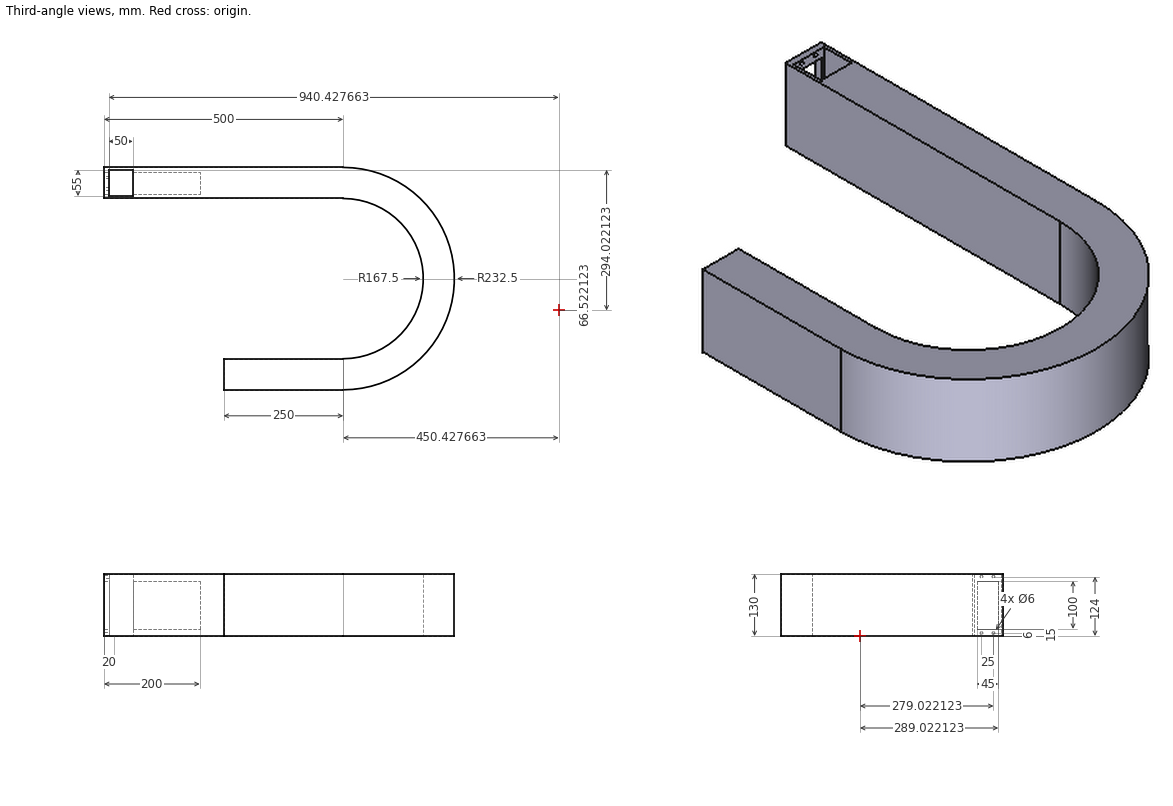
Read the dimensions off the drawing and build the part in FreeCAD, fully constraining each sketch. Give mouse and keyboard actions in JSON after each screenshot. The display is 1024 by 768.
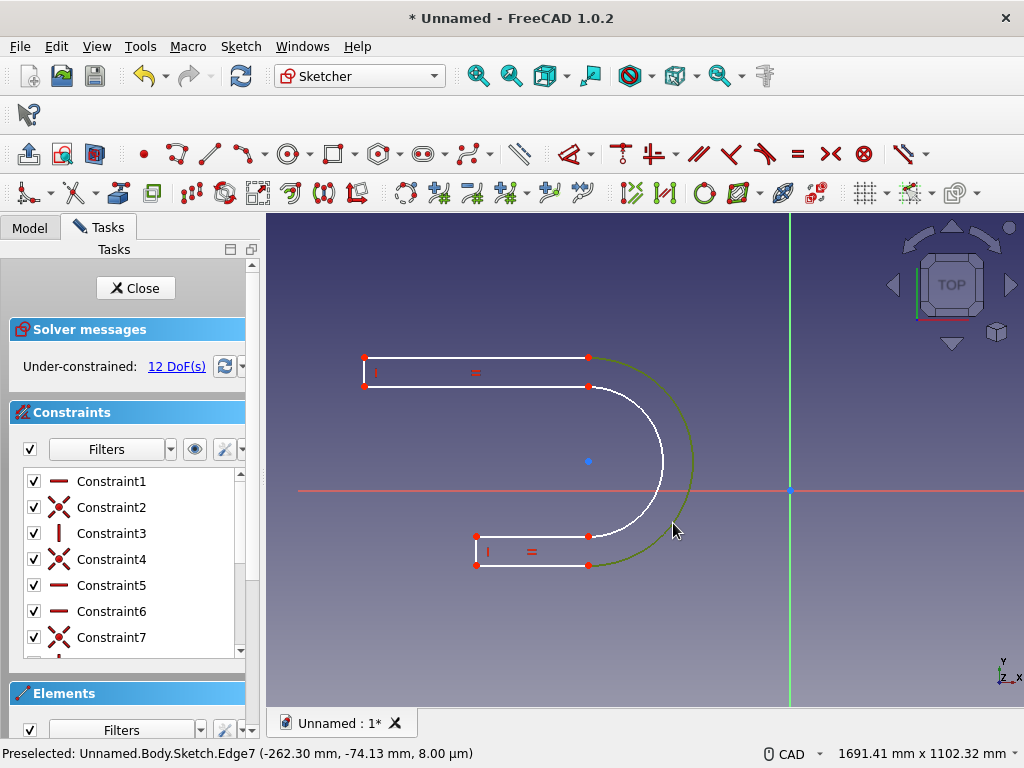
{"action": "left_click", "coordinate": [649, 506]}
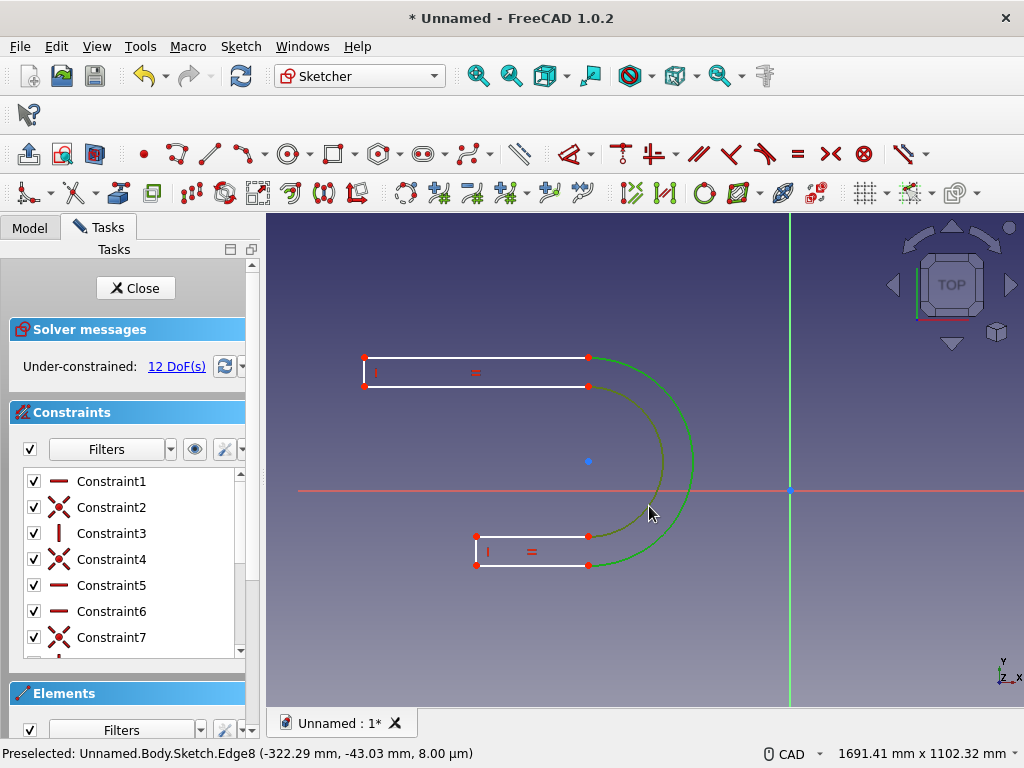
{"action": "left_click", "coordinate": [621, 154]}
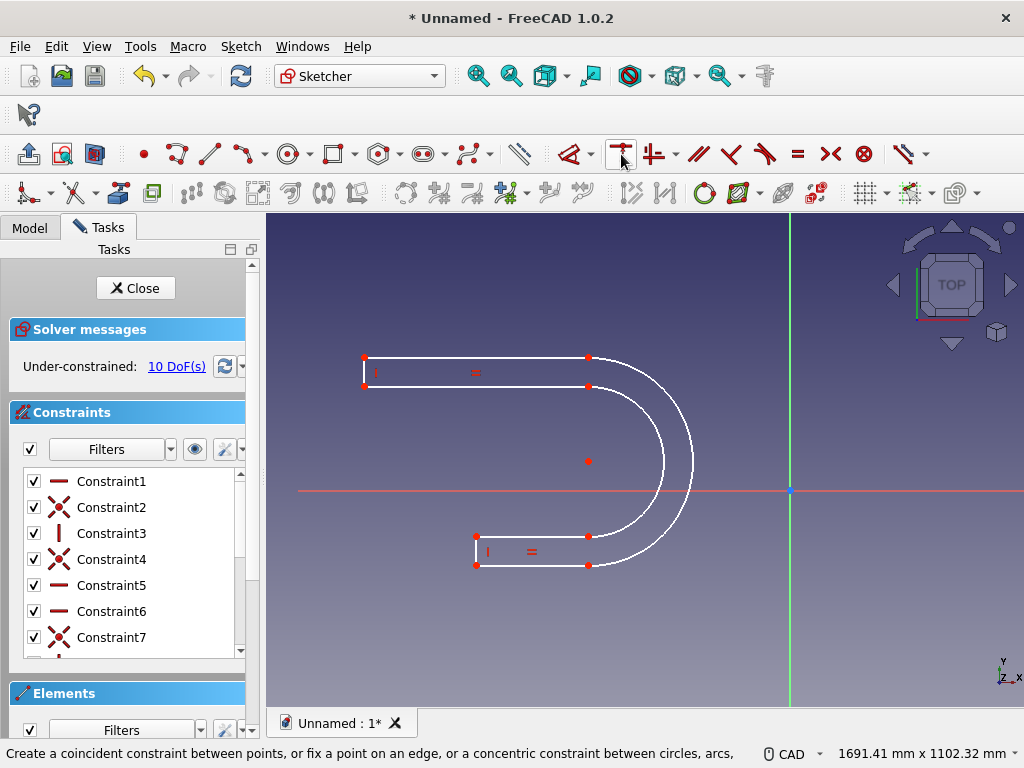
{"action": "left_click", "coordinate": [568, 154]}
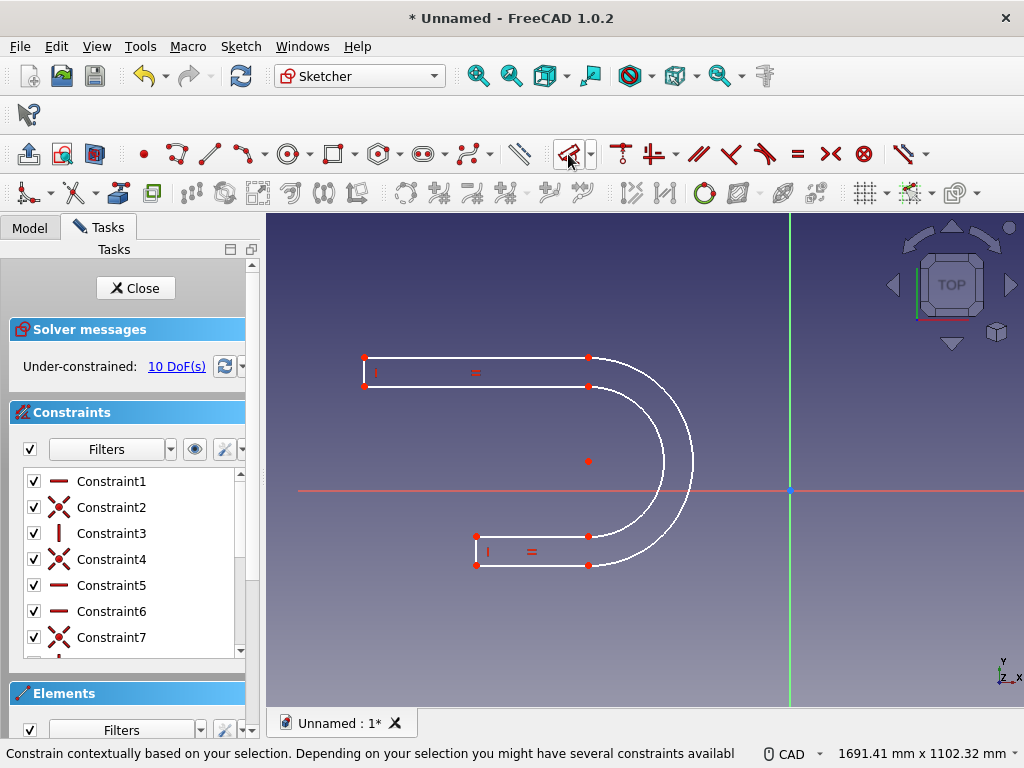
{"action": "left_click", "coordinate": [673, 523]}
{"action": "left_click", "coordinate": [699, 542]}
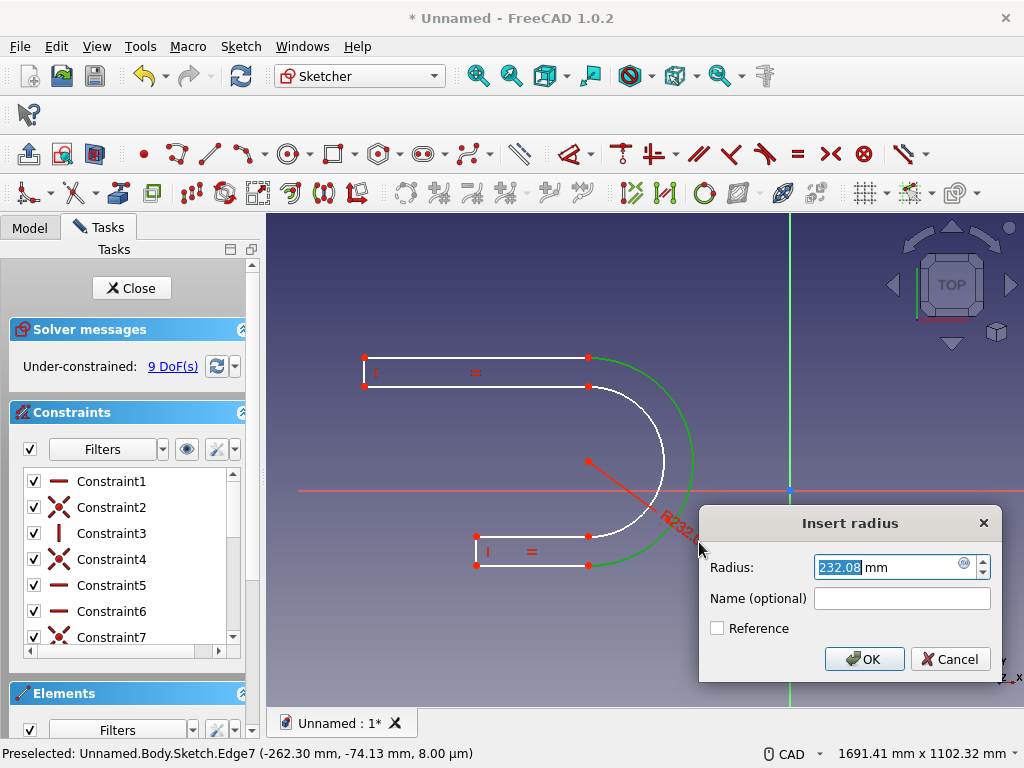
{"action": "type", "text": "232.5"}
{"action": "key", "text": "Return"}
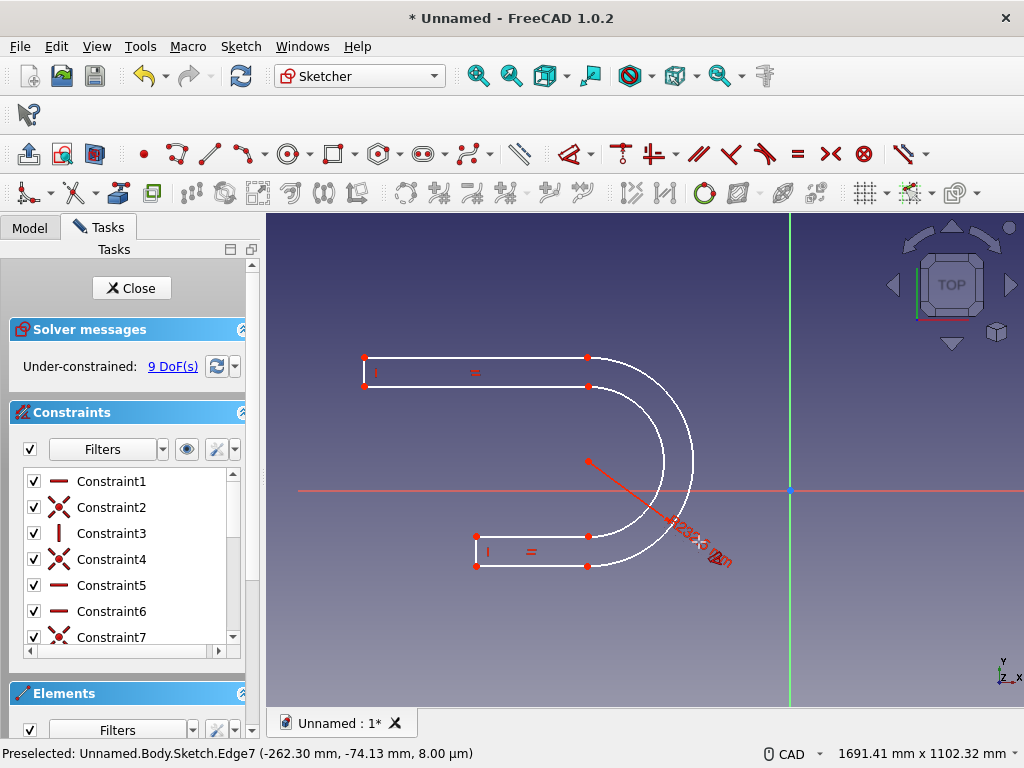
{"action": "left_click", "coordinate": [649, 506]}
{"action": "left_click", "coordinate": [644, 579]}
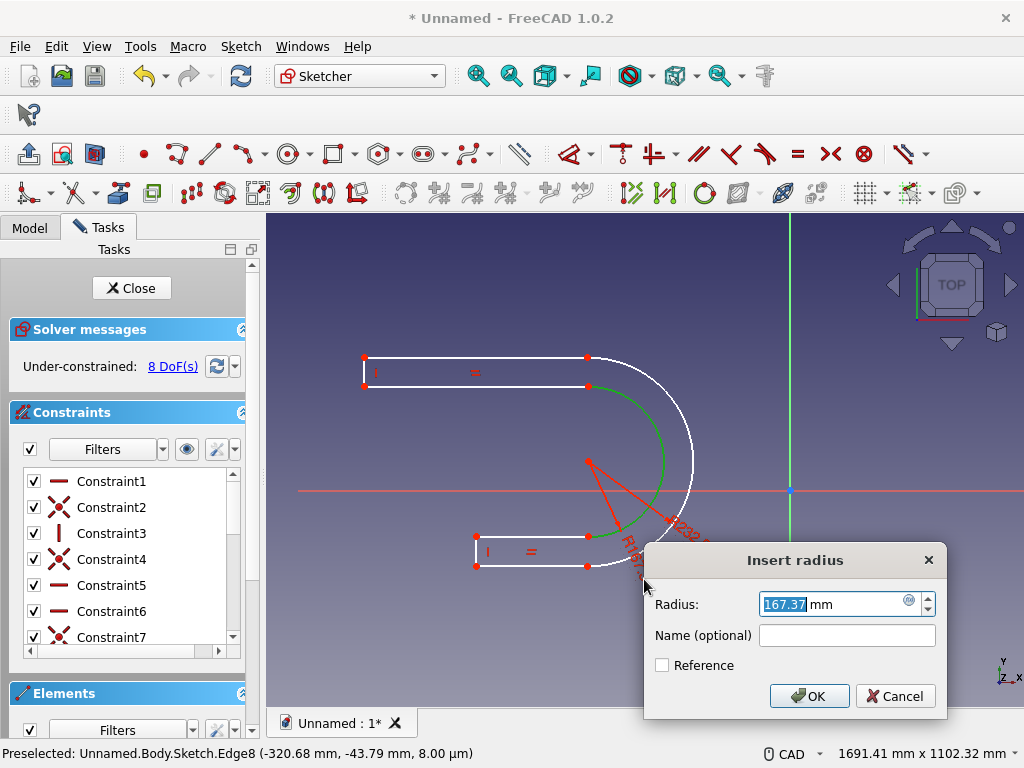
{"action": "type", "text": "167.5"}
{"action": "key", "text": "Return"}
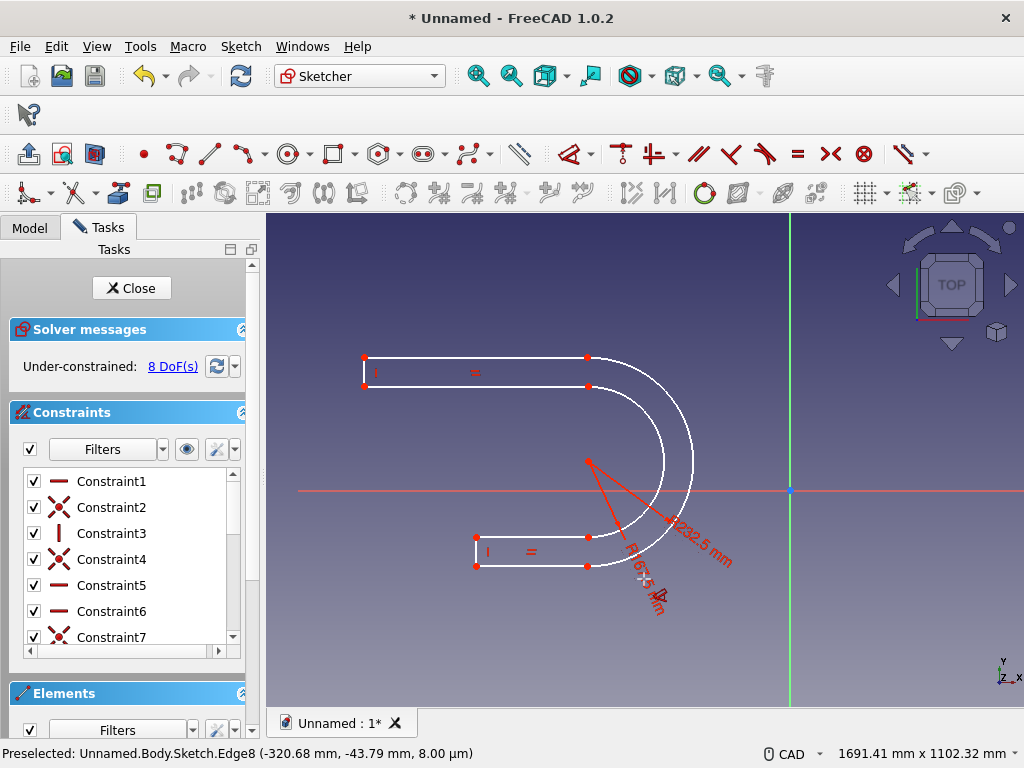
{"action": "left_click", "coordinate": [554, 537]}
{"action": "left_click", "coordinate": [532, 595]}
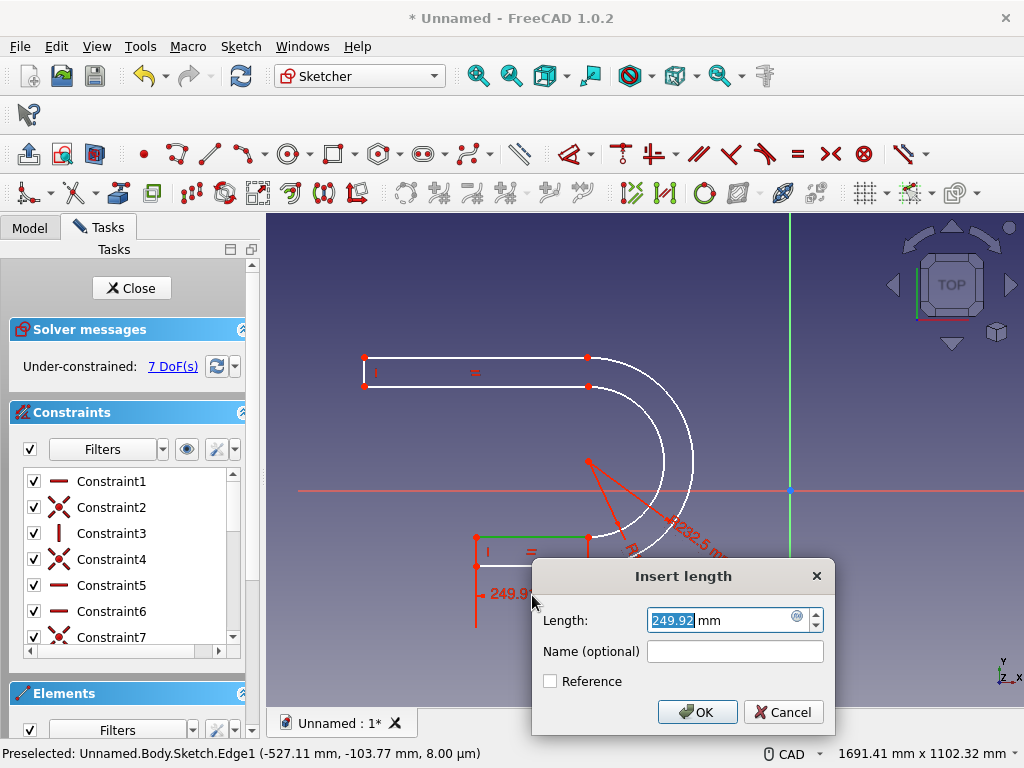
{"action": "type", "text": "250"}
{"action": "key", "text": "Return"}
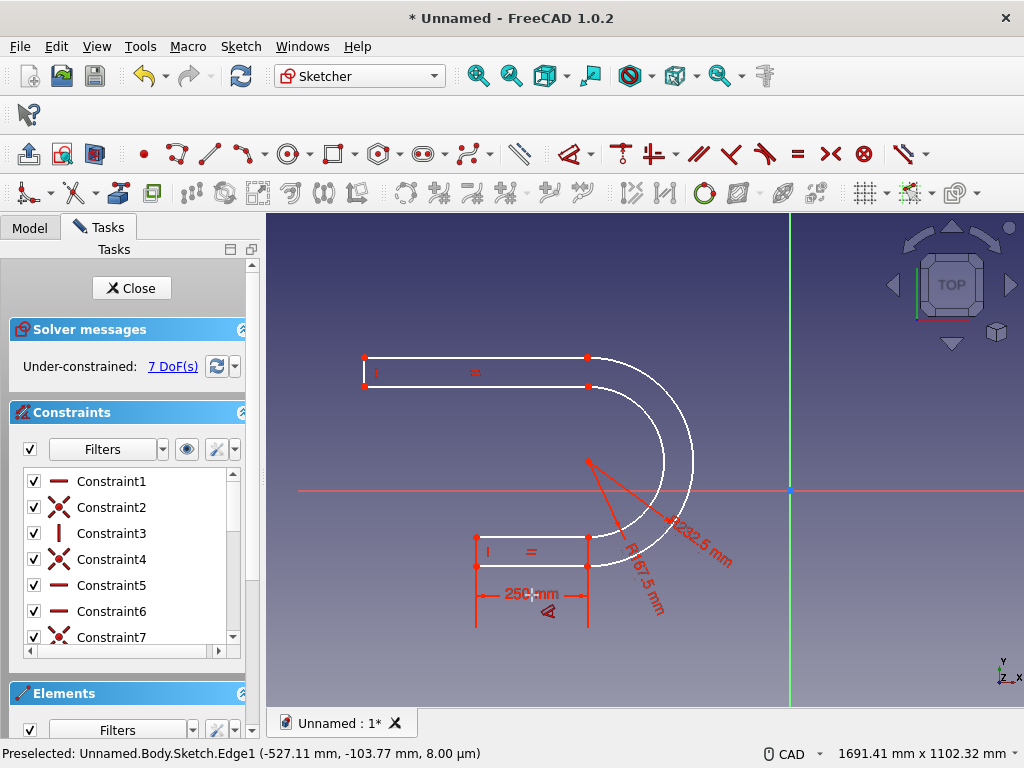
{"action": "left_click", "coordinate": [510, 566]}
{"action": "left_click", "coordinate": [532, 624]}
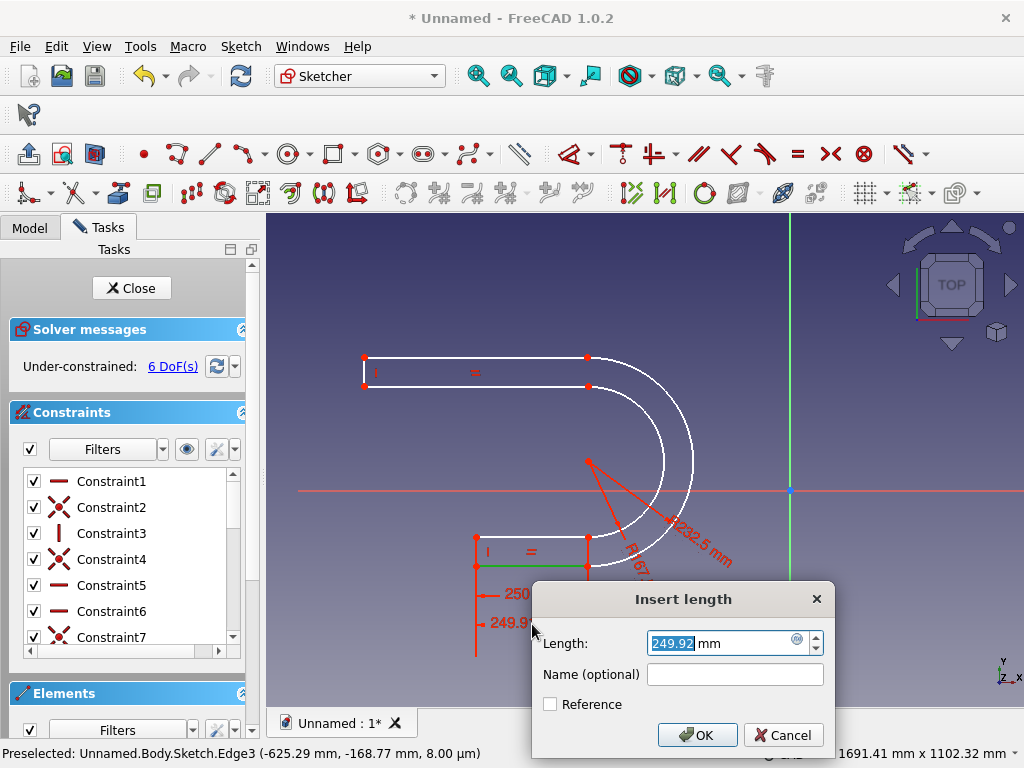
{"action": "type", "text": "250"}
{"action": "key", "text": "Return"}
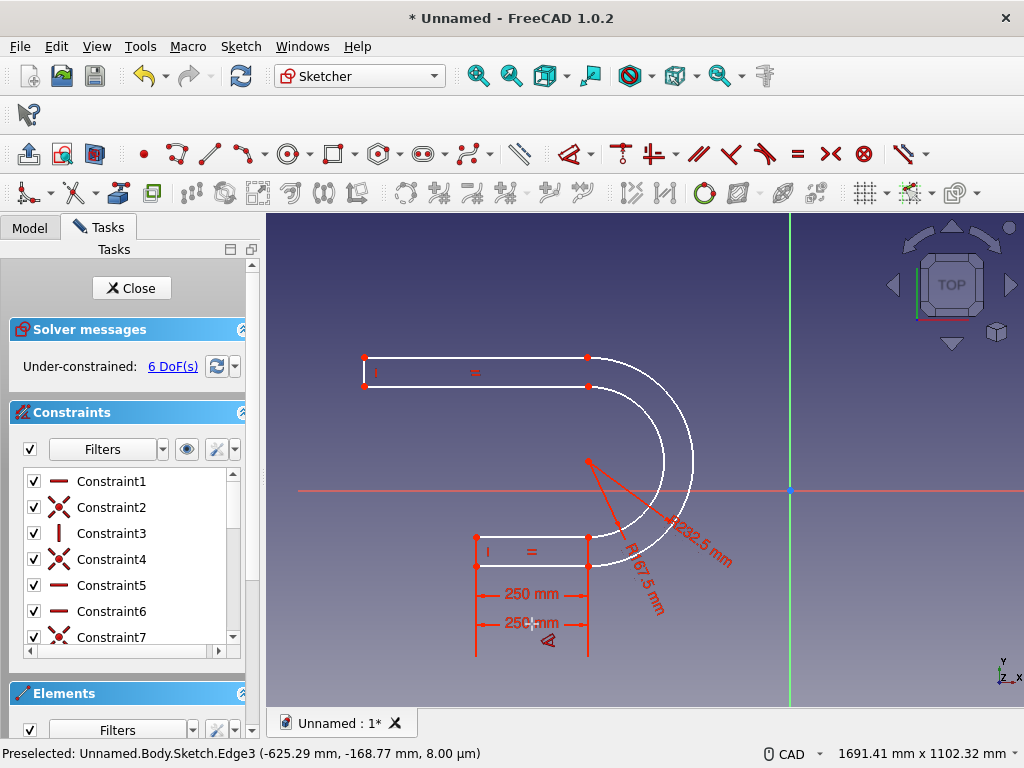
{"action": "left_click", "coordinate": [521, 358]}
{"action": "left_click", "coordinate": [476, 324]}